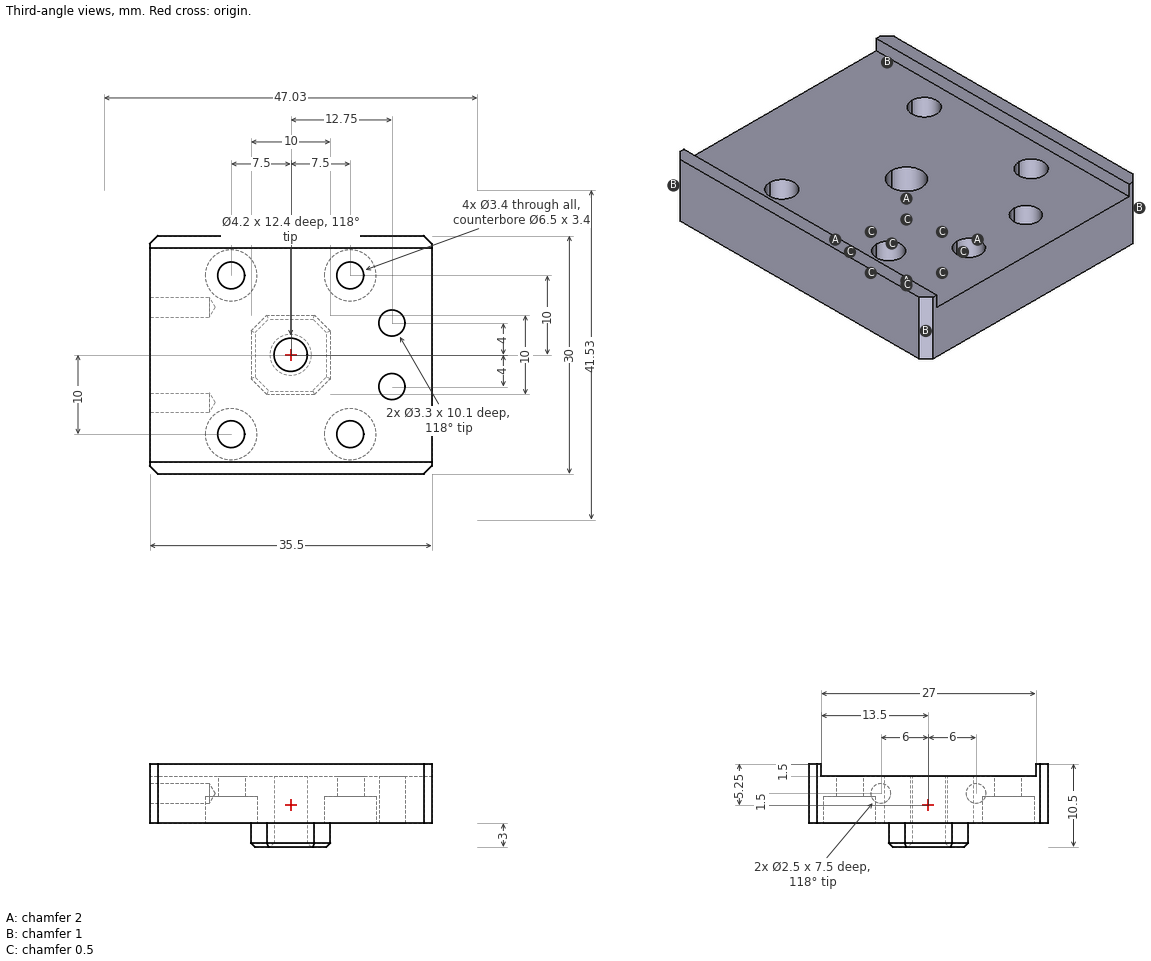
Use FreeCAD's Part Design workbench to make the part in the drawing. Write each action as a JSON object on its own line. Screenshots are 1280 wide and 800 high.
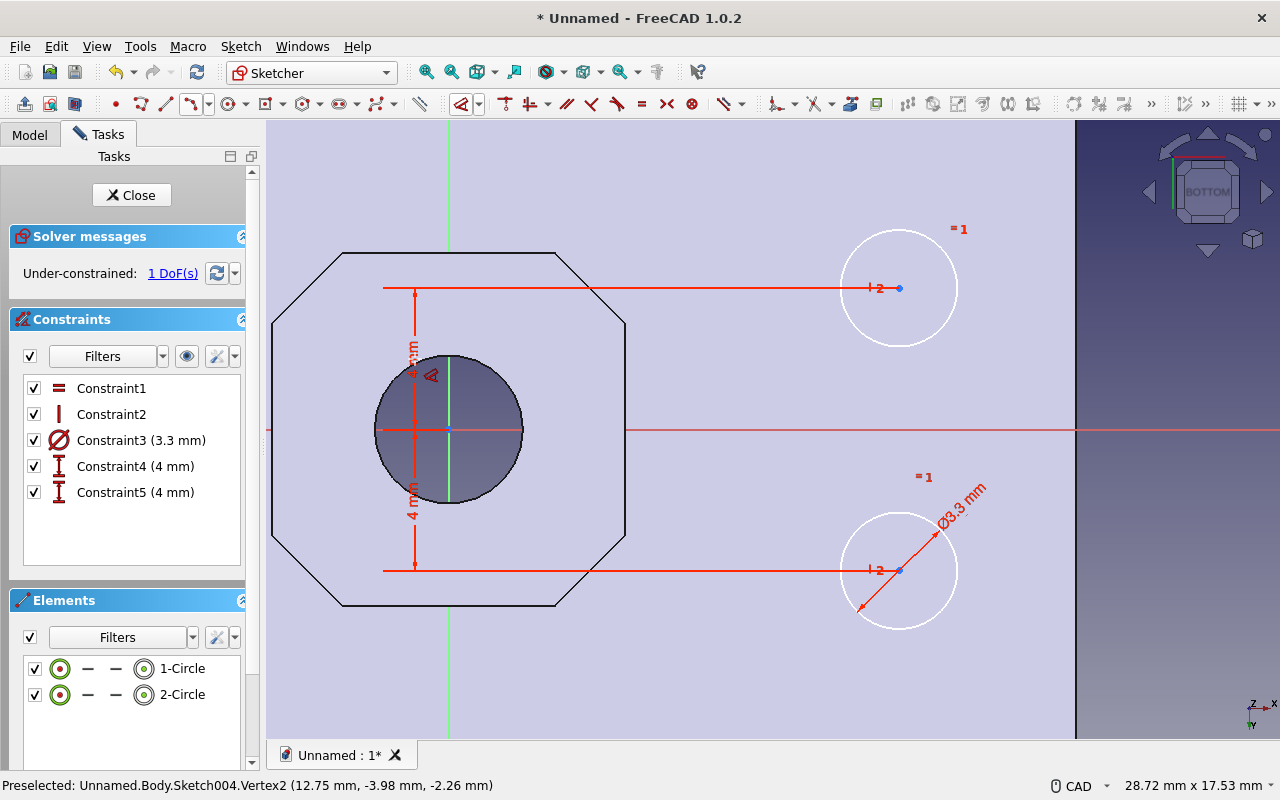
{"action": "left_click", "coordinate": [899, 571]}
{"action": "left_click", "coordinate": [674, 605]}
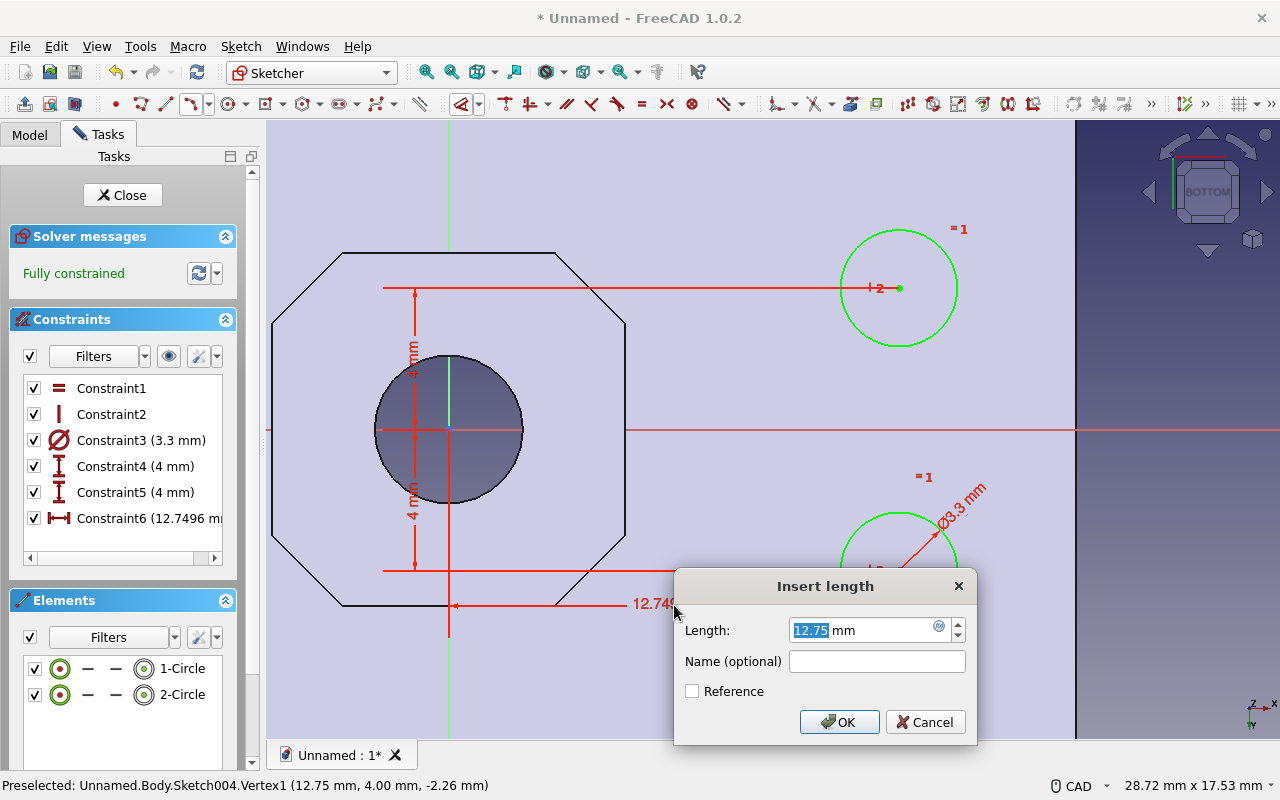
{"action": "type", "text": "12.75"}
{"action": "key", "text": "Return"}
{"action": "key", "text": "Escape"}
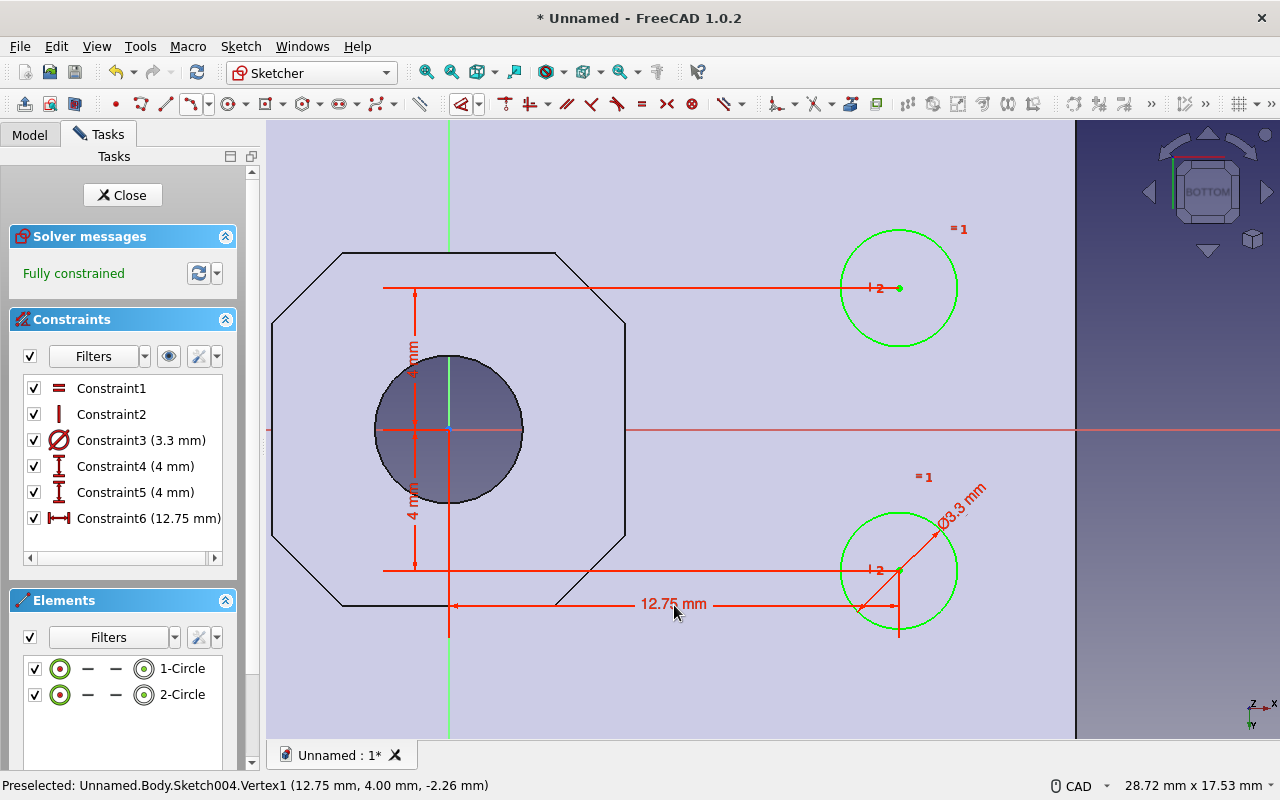
{"action": "left_click", "coordinate": [123, 195]}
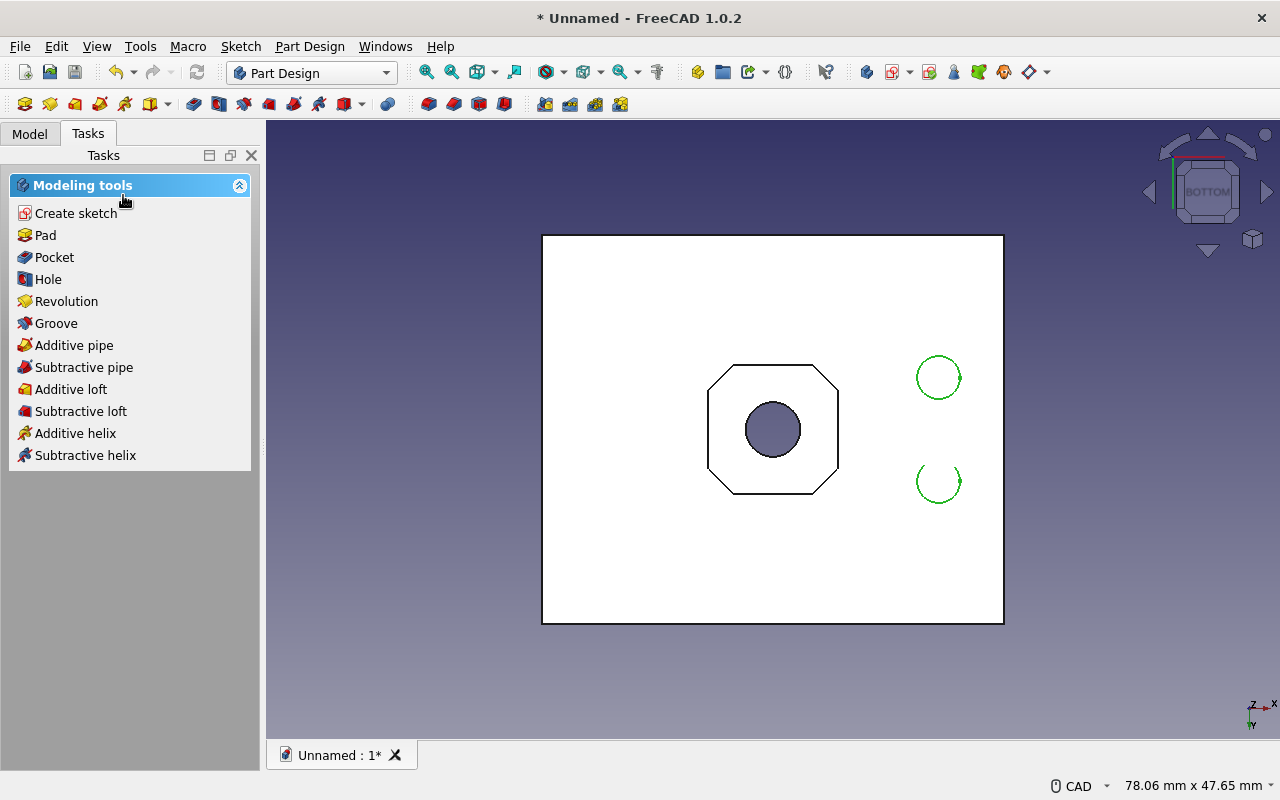
{"action": "left_click", "coordinate": [219, 104]}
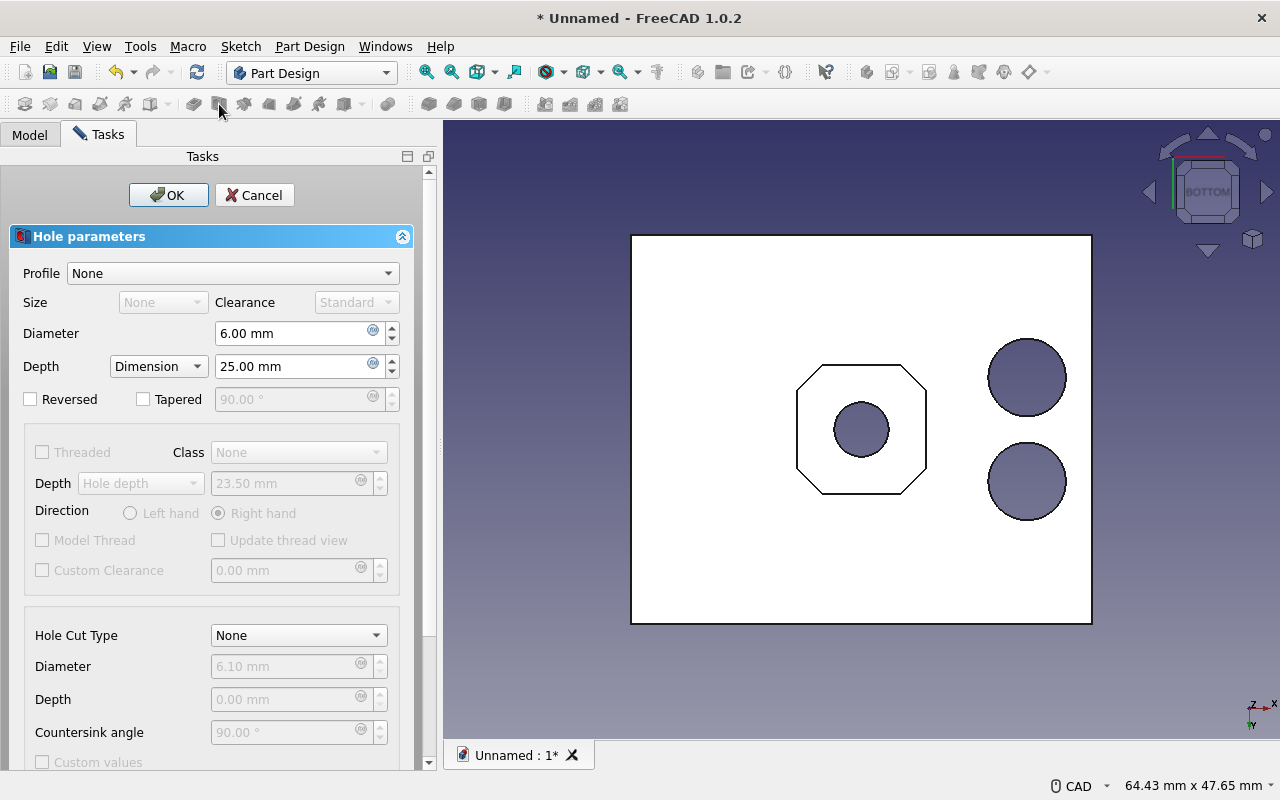
{"action": "triple_click", "coordinate": [300, 334]}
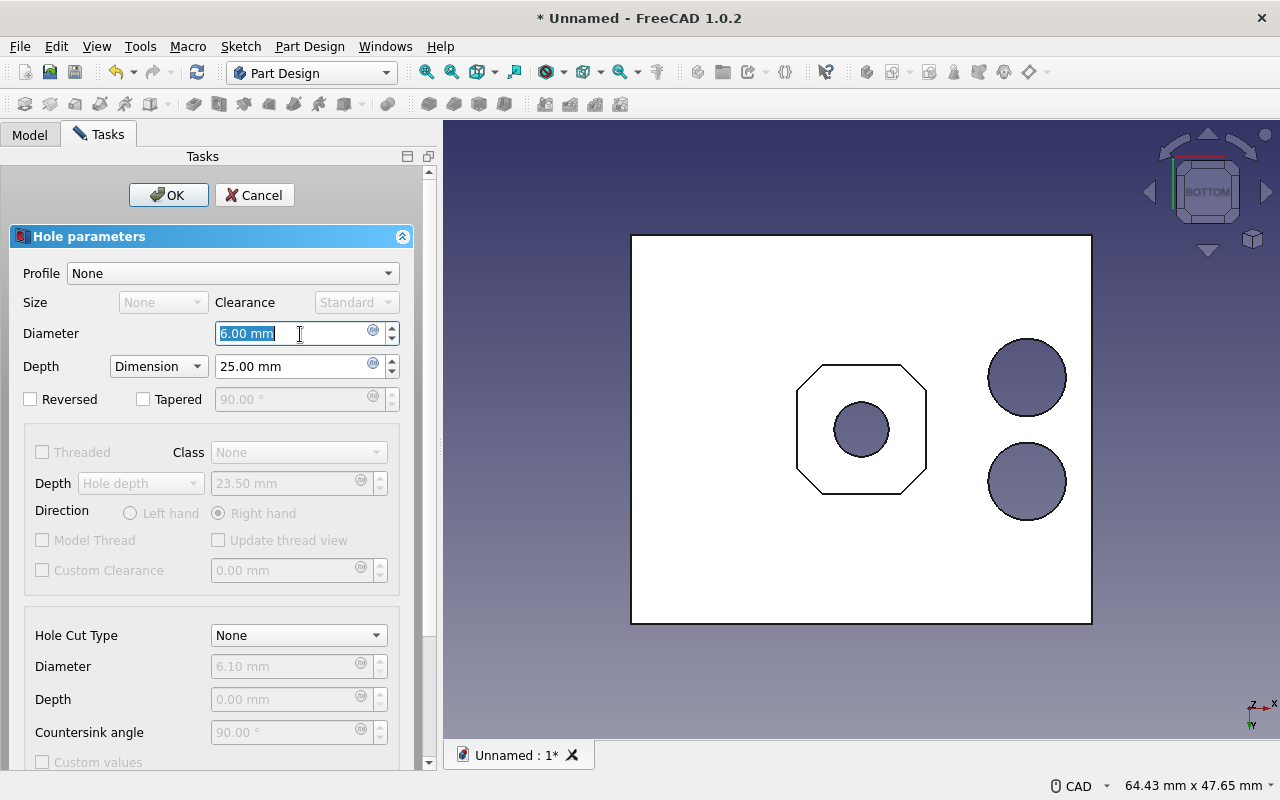
{"action": "type", "text": "3.3"}
{"action": "key", "text": "Tab"}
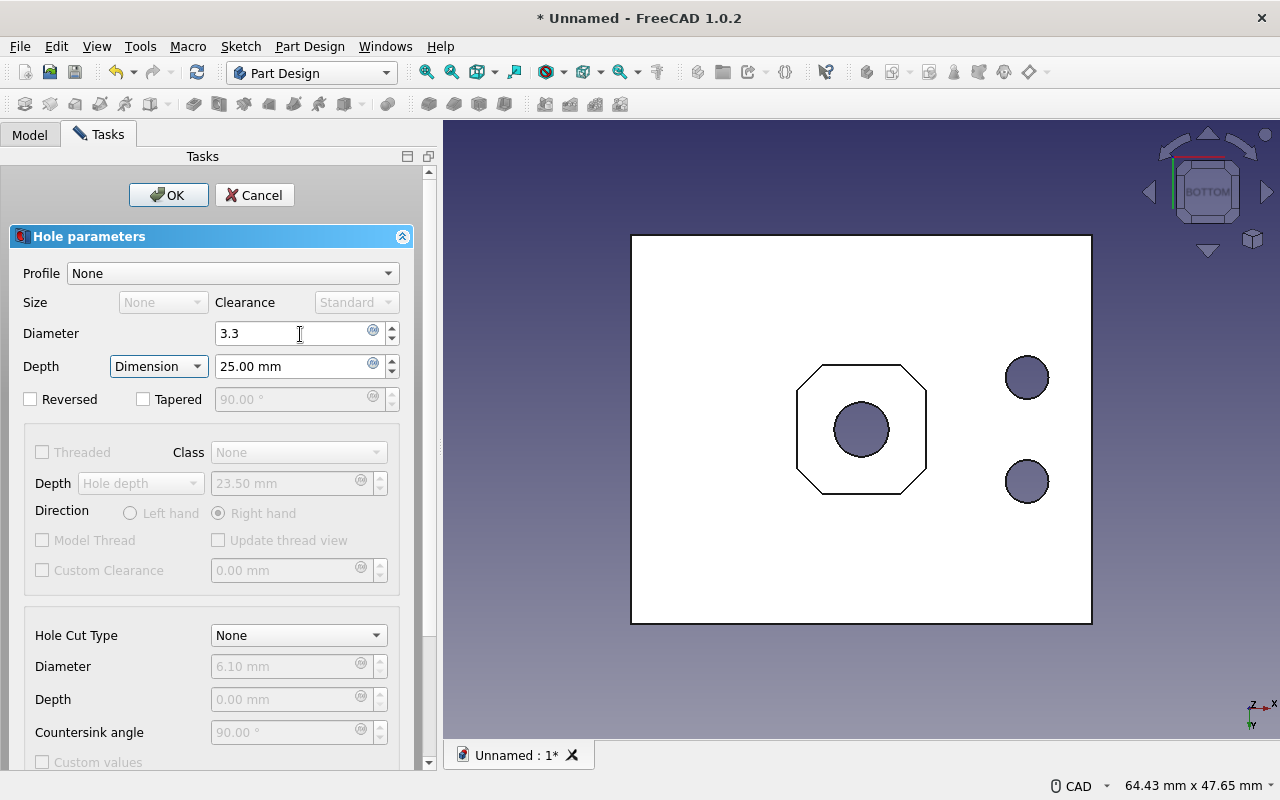
{"action": "triple_click", "coordinate": [300, 366]}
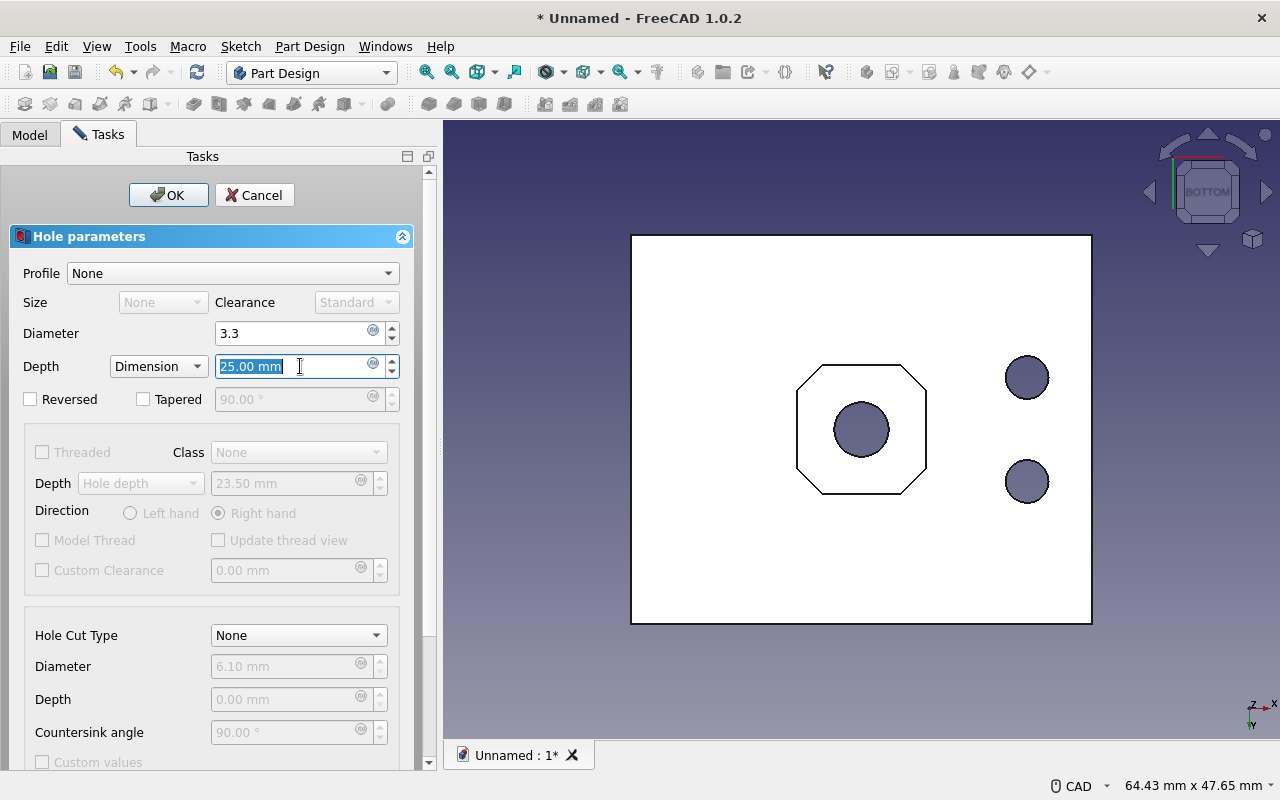
{"action": "type", "text": "10.1"}
{"action": "key", "text": "Tab"}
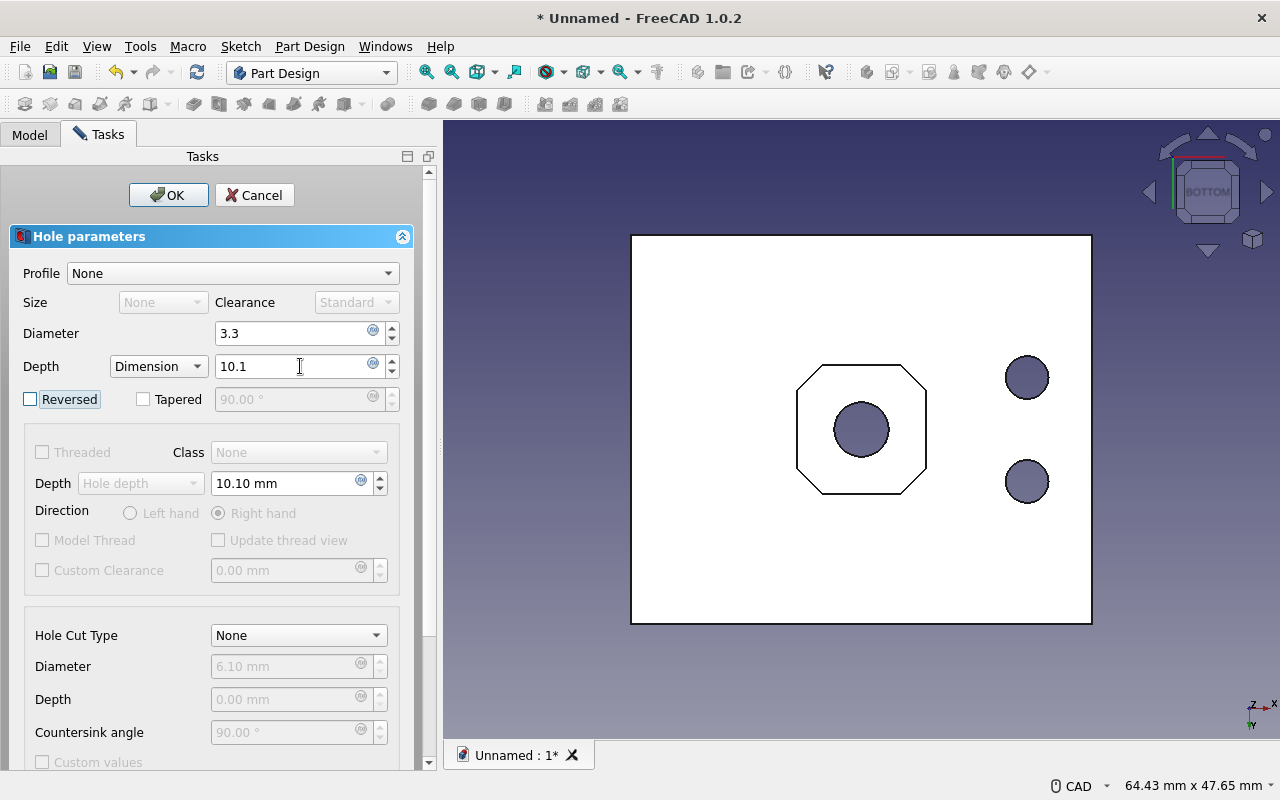
{"action": "left_click", "coordinate": [169, 195]}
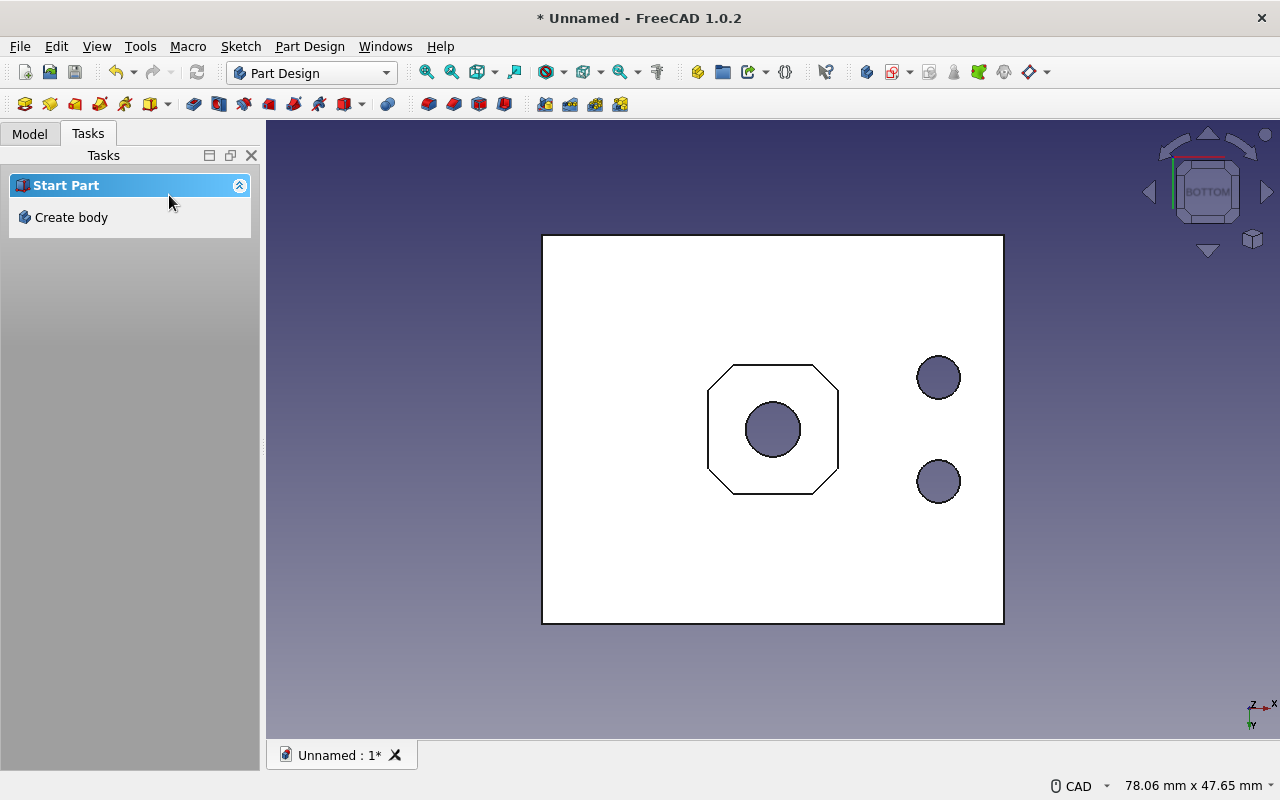
{"action": "key", "text": "0"}